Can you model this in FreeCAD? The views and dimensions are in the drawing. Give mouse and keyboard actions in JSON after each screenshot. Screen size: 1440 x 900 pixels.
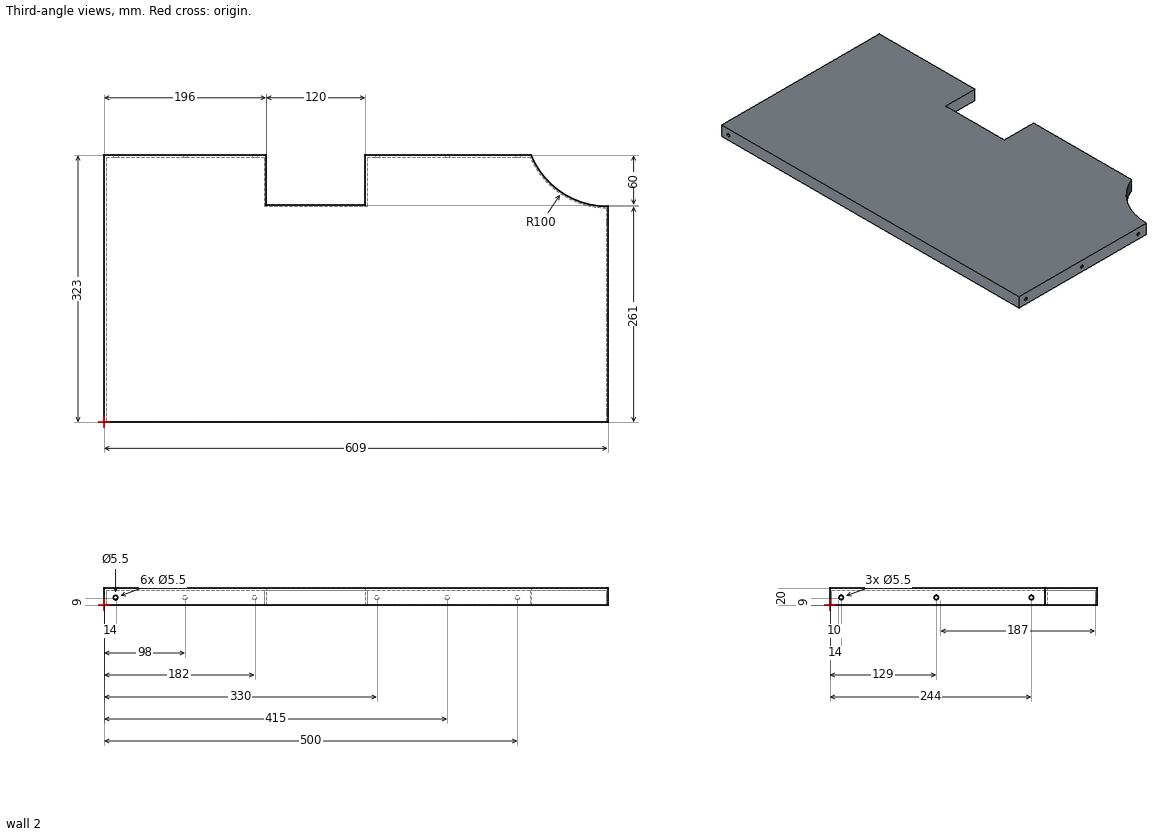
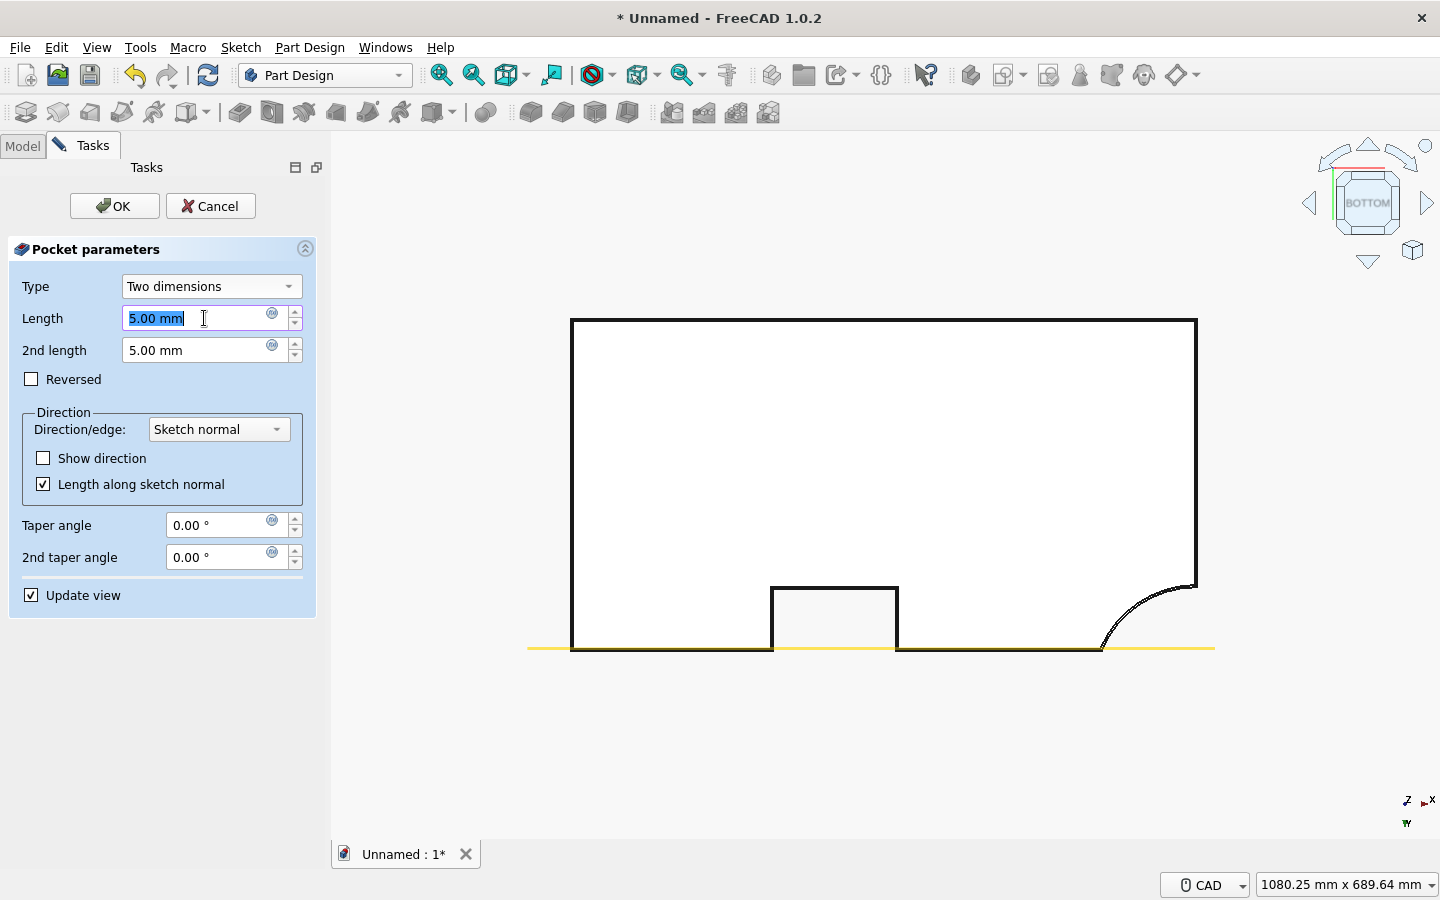
{"action": "type", "text": "187"}
{"action": "key", "text": "Tab"}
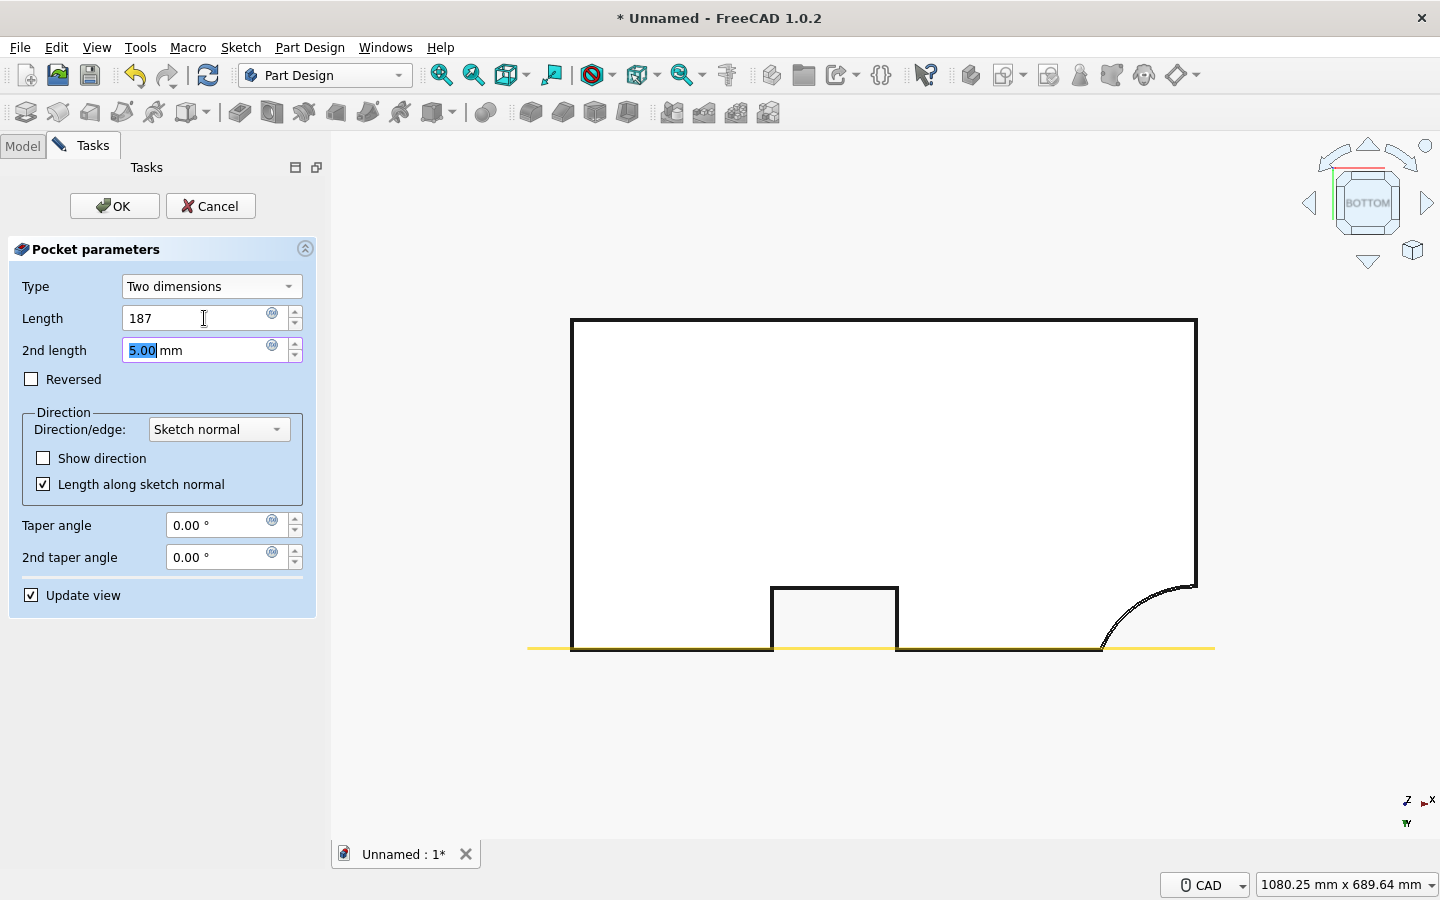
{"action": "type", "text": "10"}
{"action": "key", "text": "Tab"}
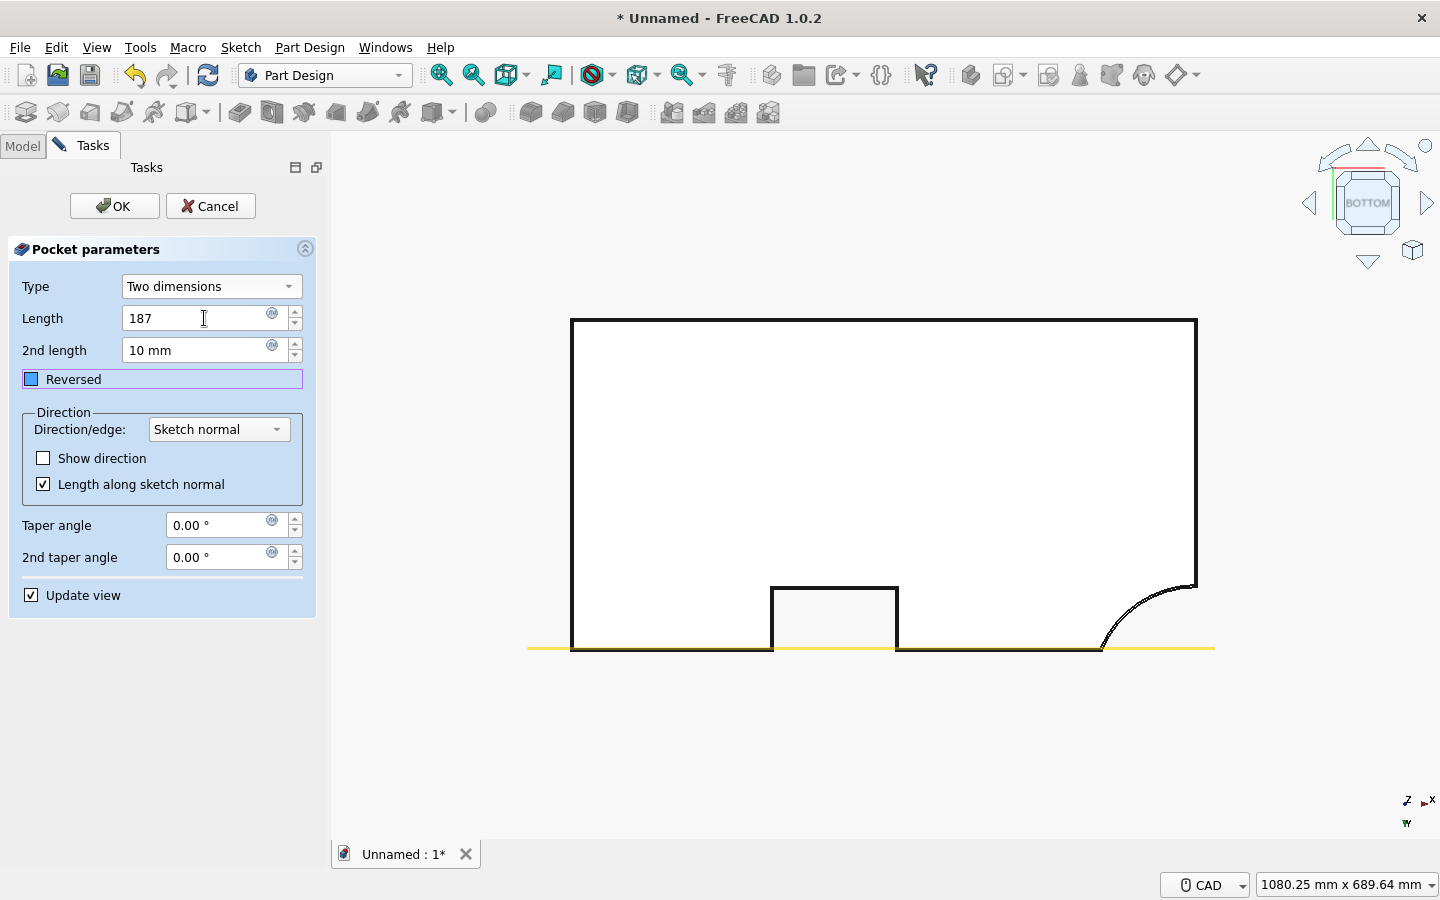
{"action": "left_click", "coordinate": [30, 379]}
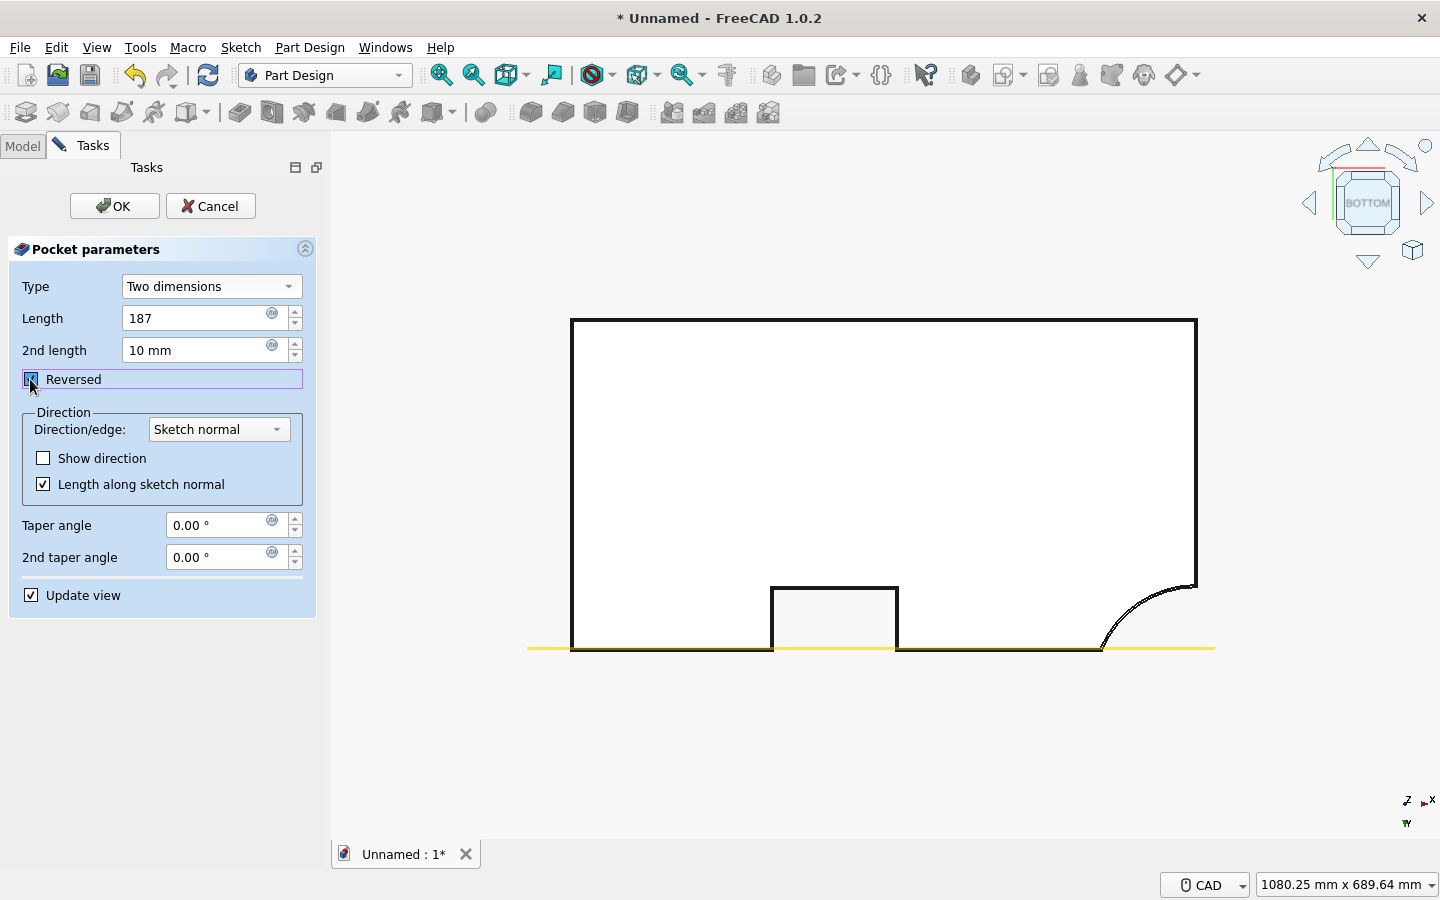
{"action": "left_click", "coordinate": [115, 206]}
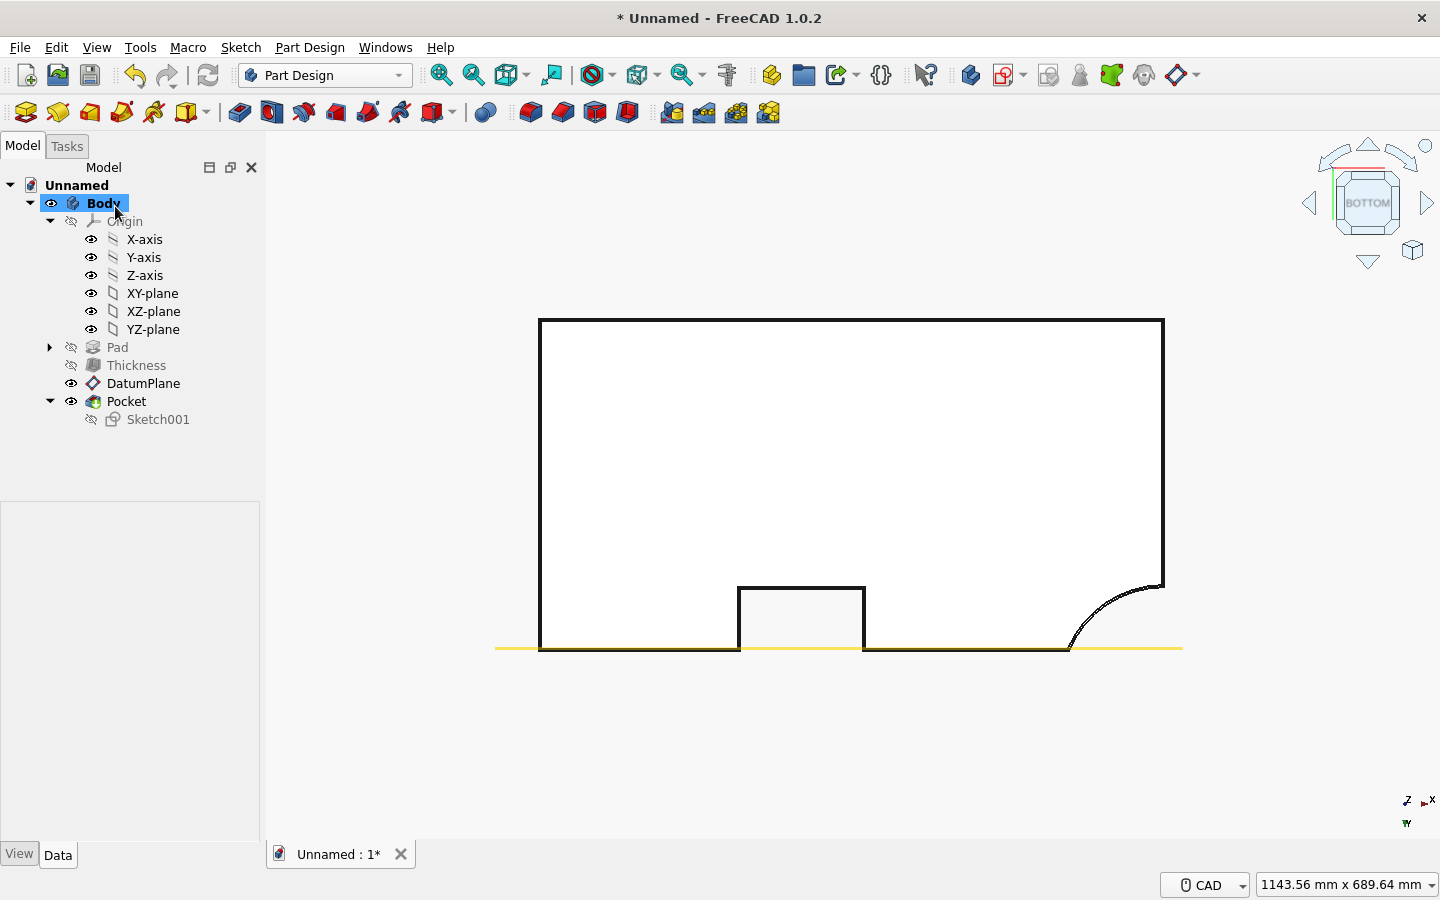
{"action": "left_click", "coordinate": [116, 383]}
{"action": "key", "text": "space"}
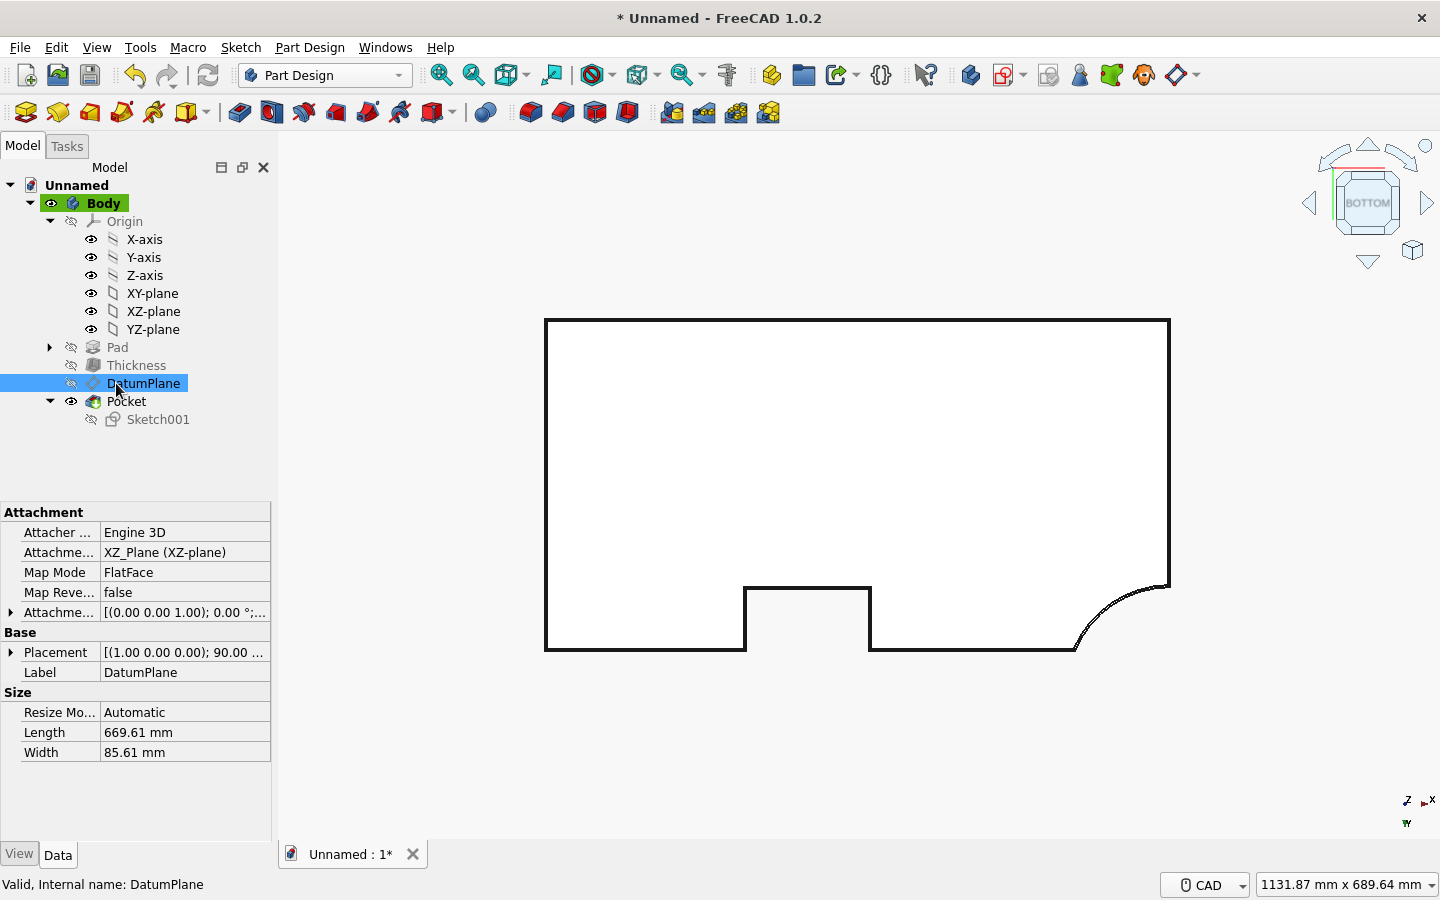
{"action": "left_click", "coordinate": [318, 799]}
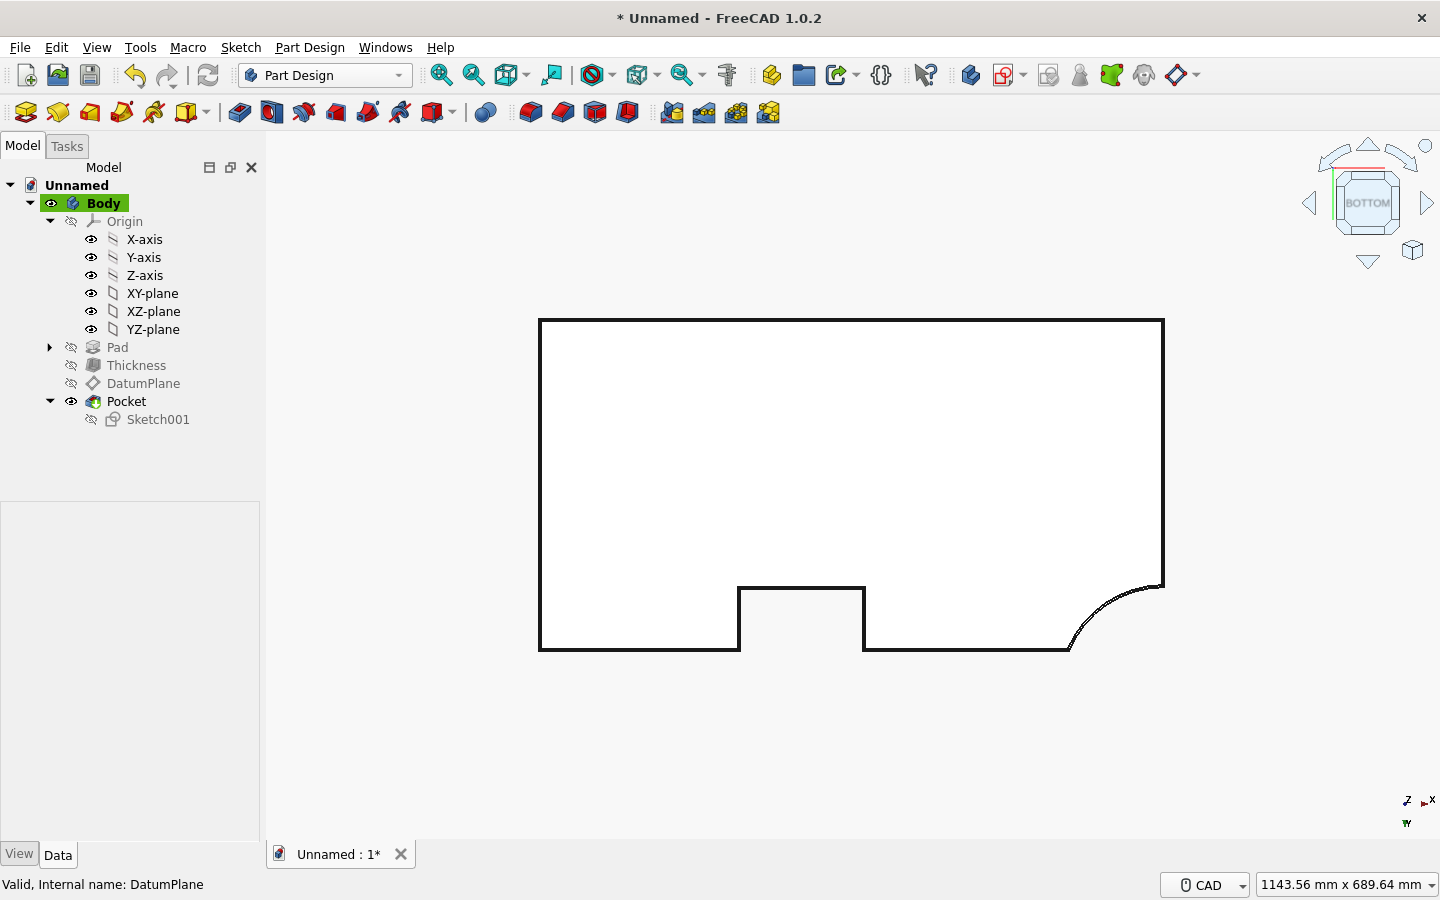
{"action": "left_click", "coordinate": [1004, 76]}